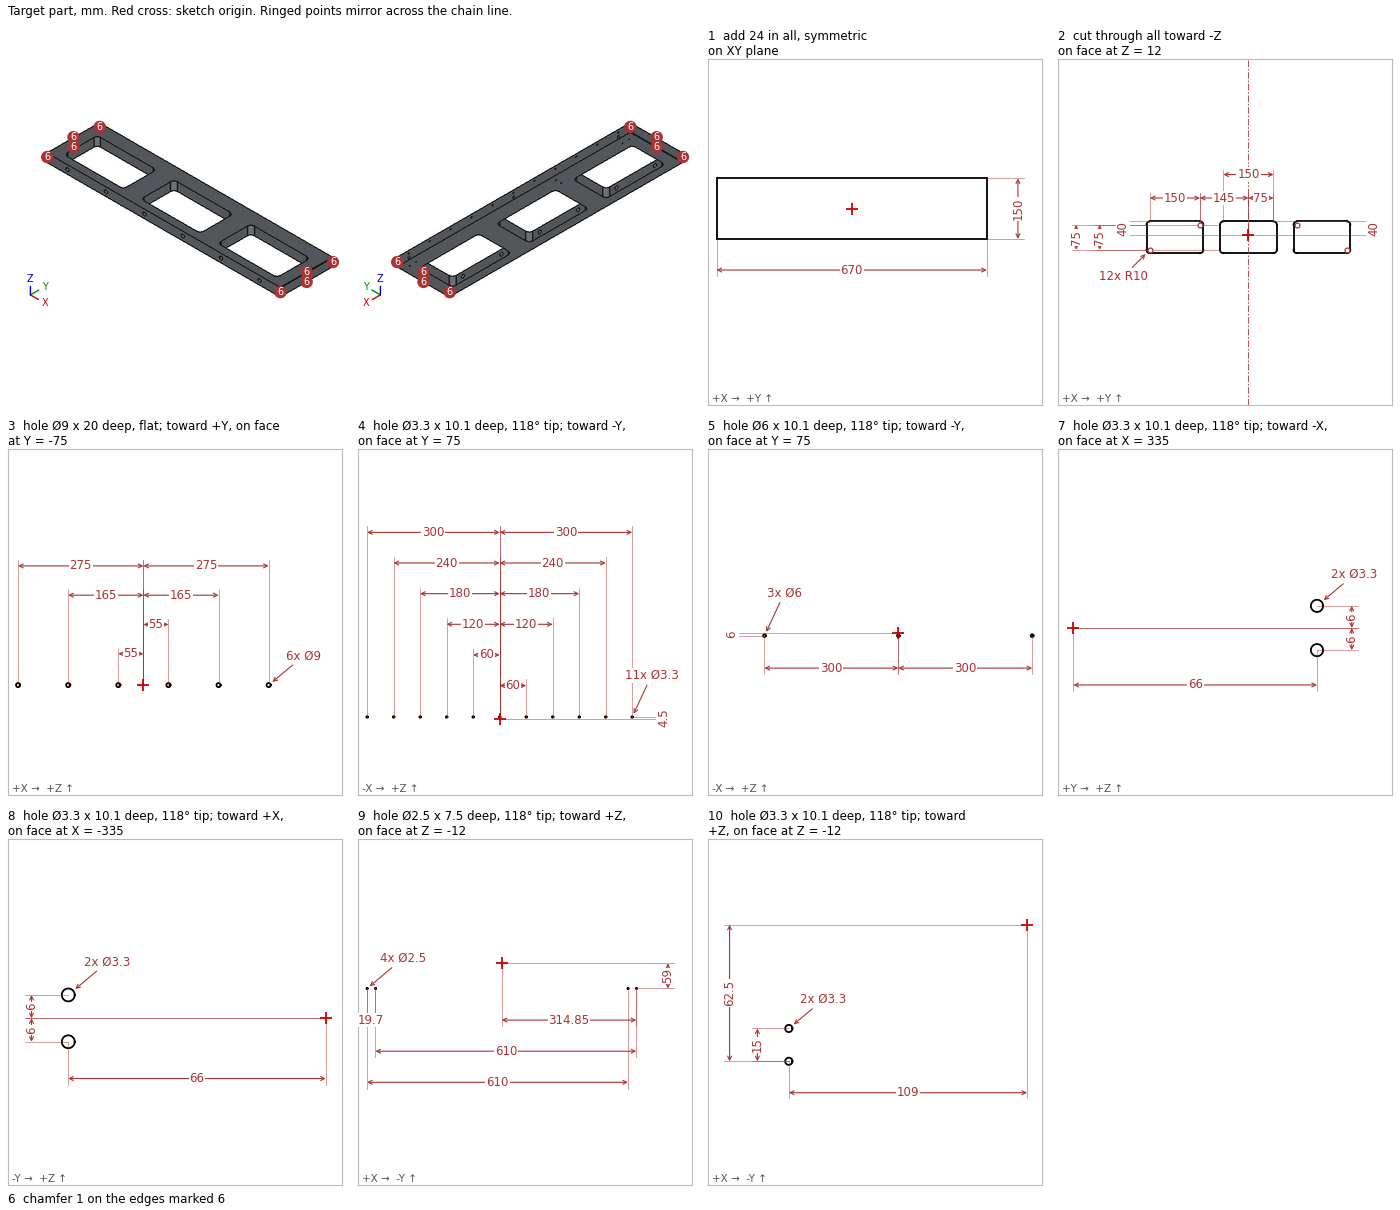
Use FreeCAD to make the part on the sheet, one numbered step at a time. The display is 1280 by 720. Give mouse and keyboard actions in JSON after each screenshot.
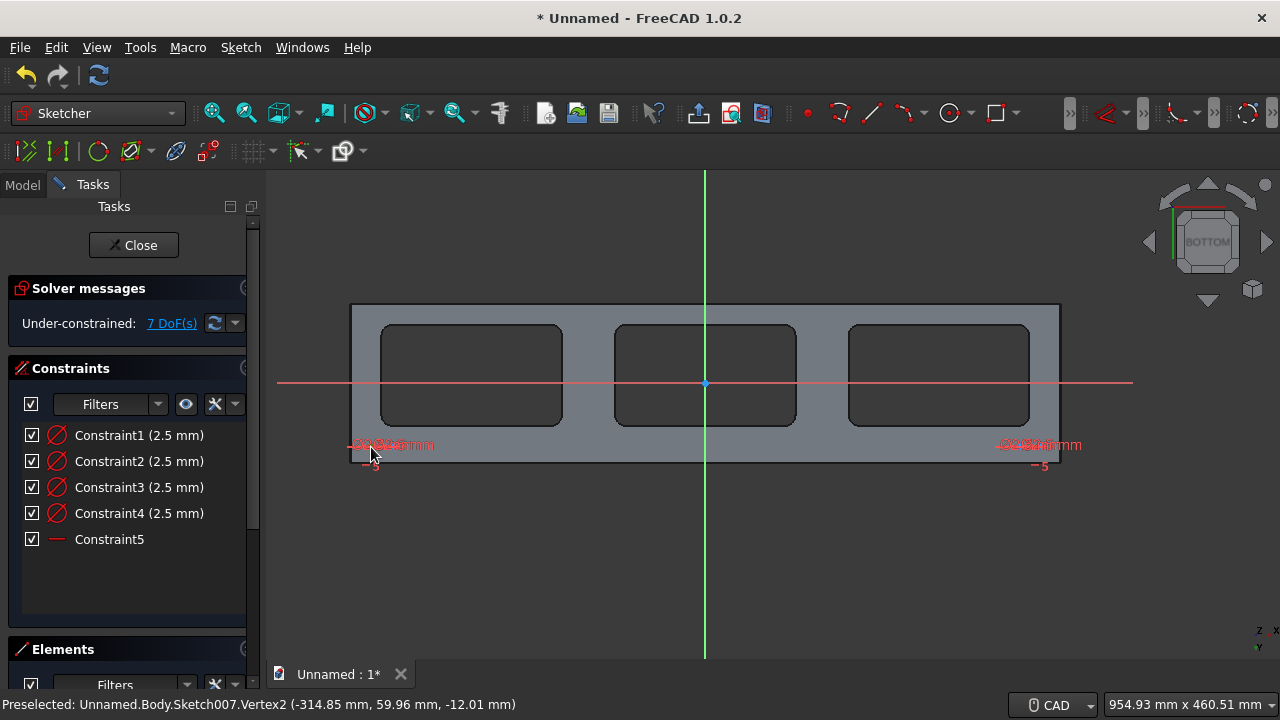
{"action": "left_click", "coordinate": [392, 447]}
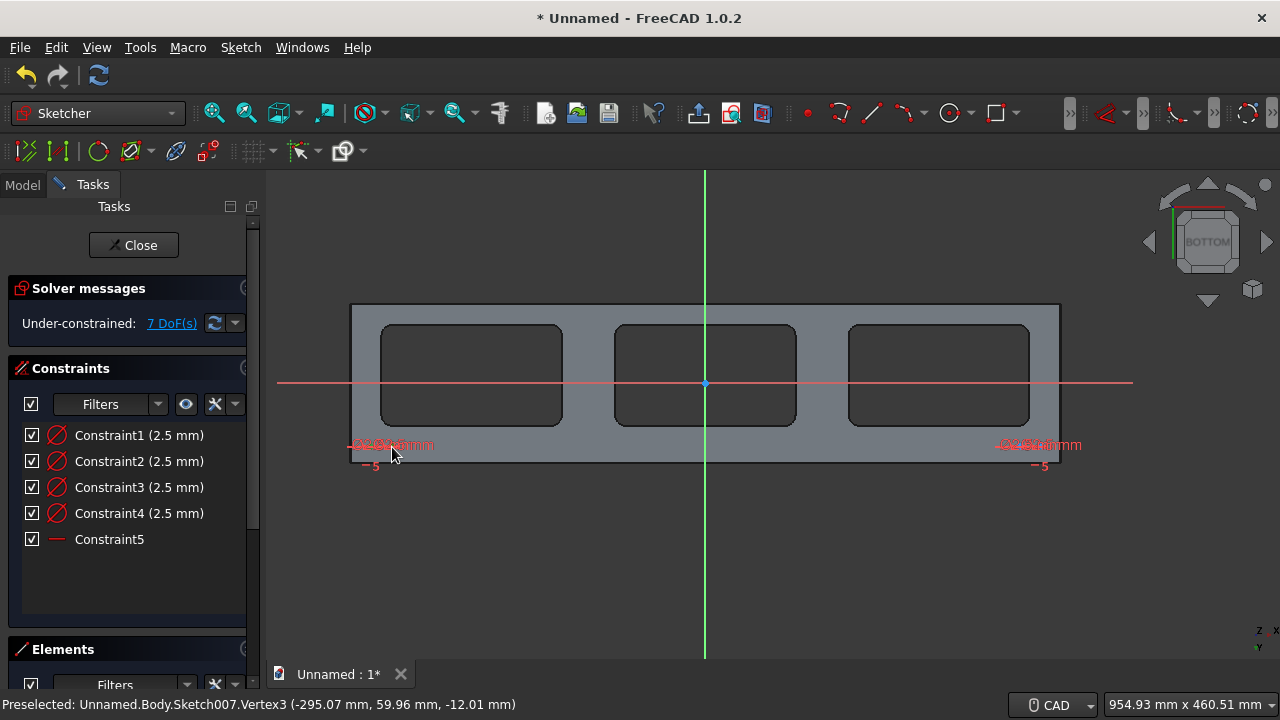
{"action": "key", "text": "h"}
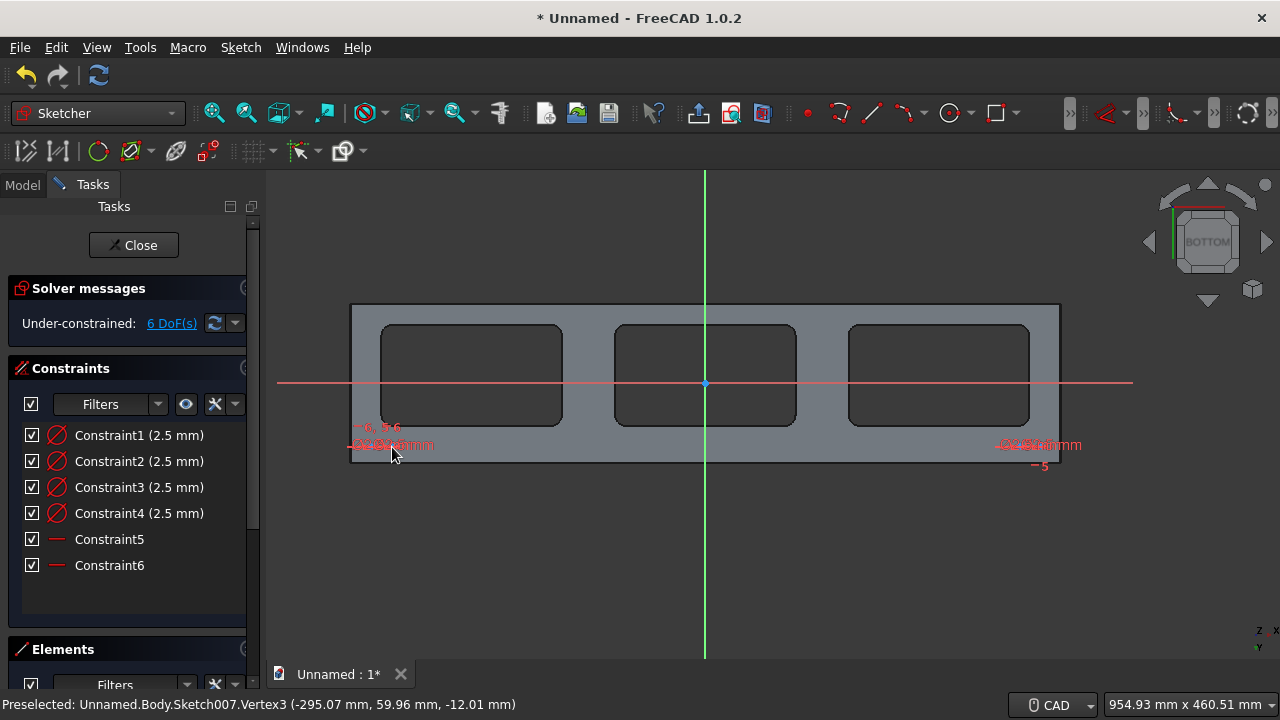
{"action": "left_click", "coordinate": [1040, 447]}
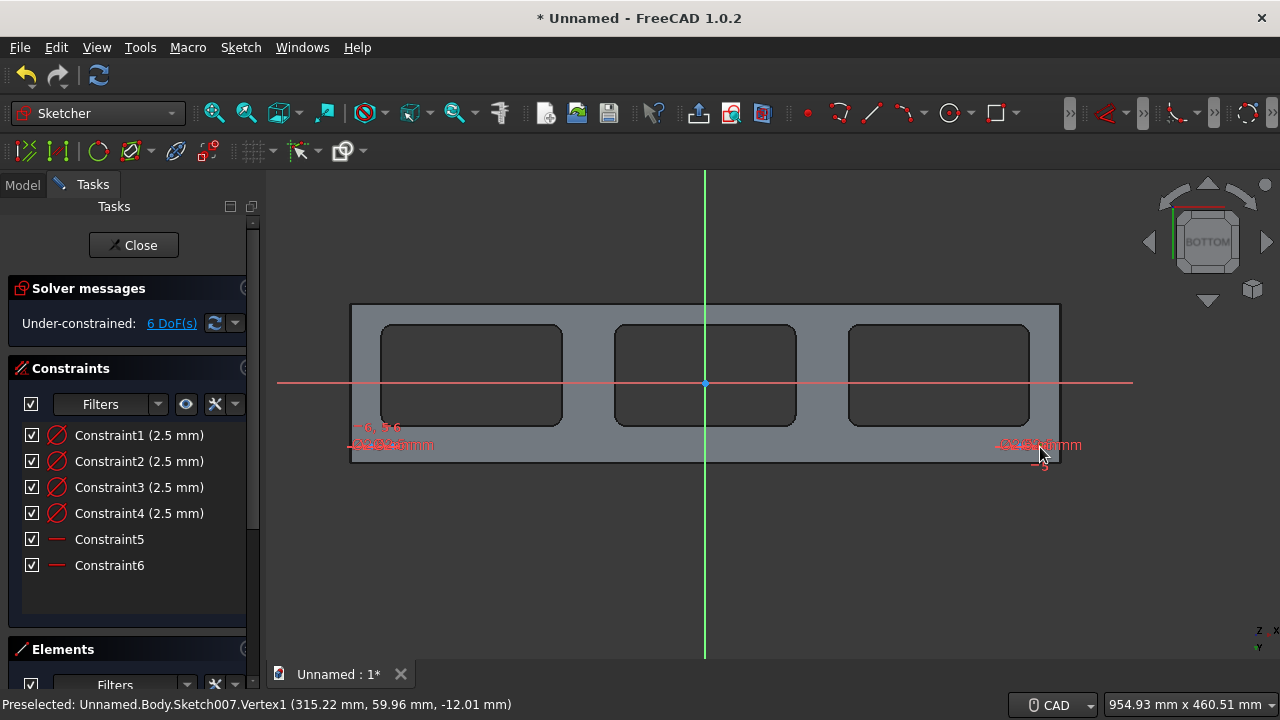
{"action": "left_click", "coordinate": [1019, 447]}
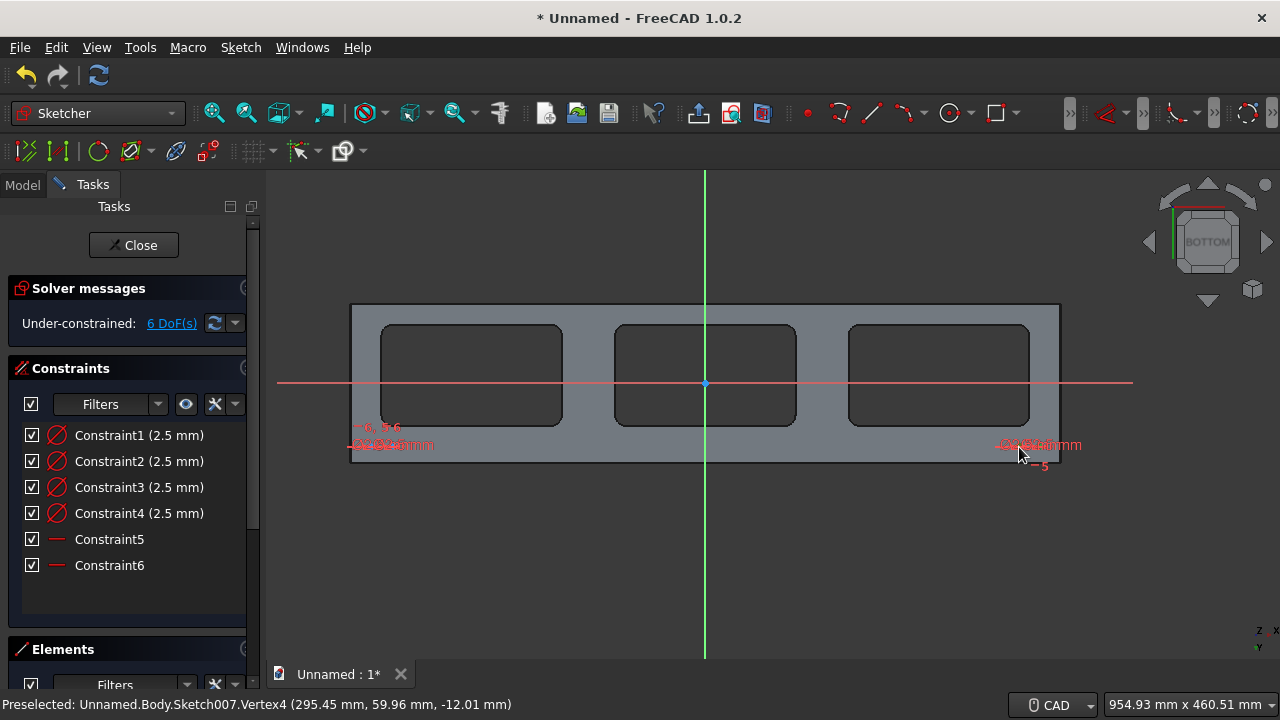
{"action": "key", "text": "h"}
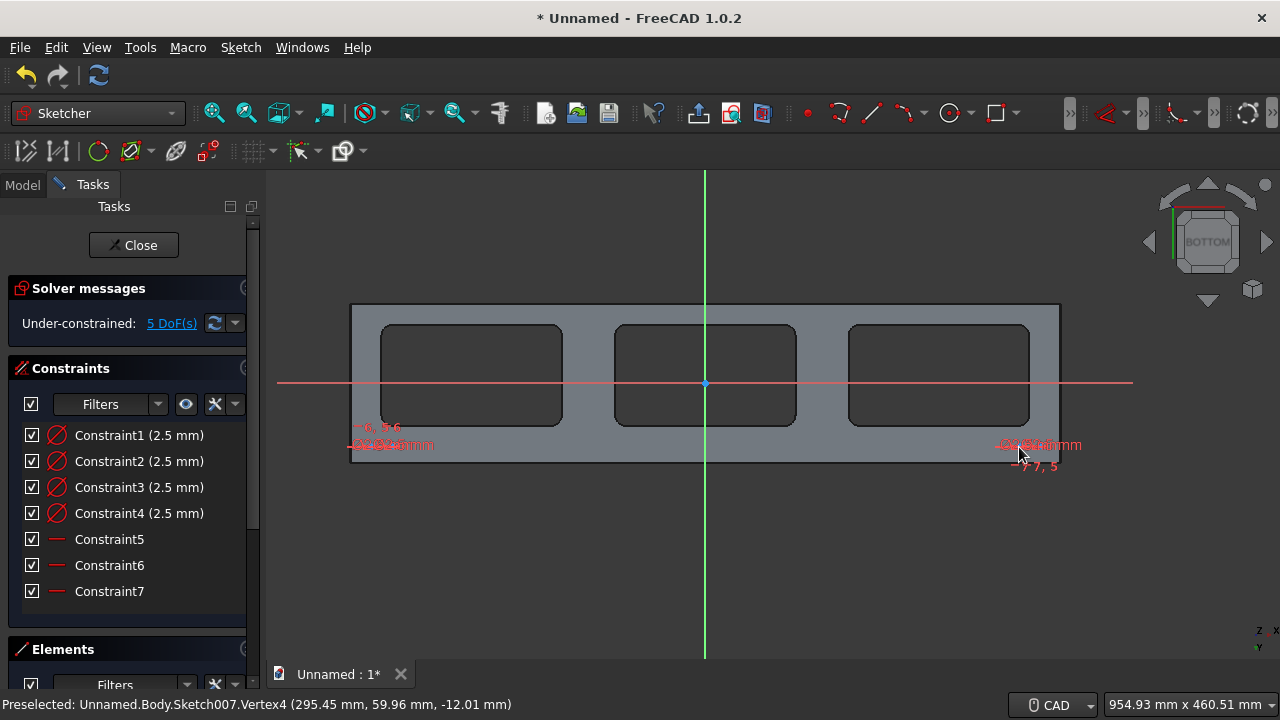
{"action": "left_click", "coordinate": [1106, 114]}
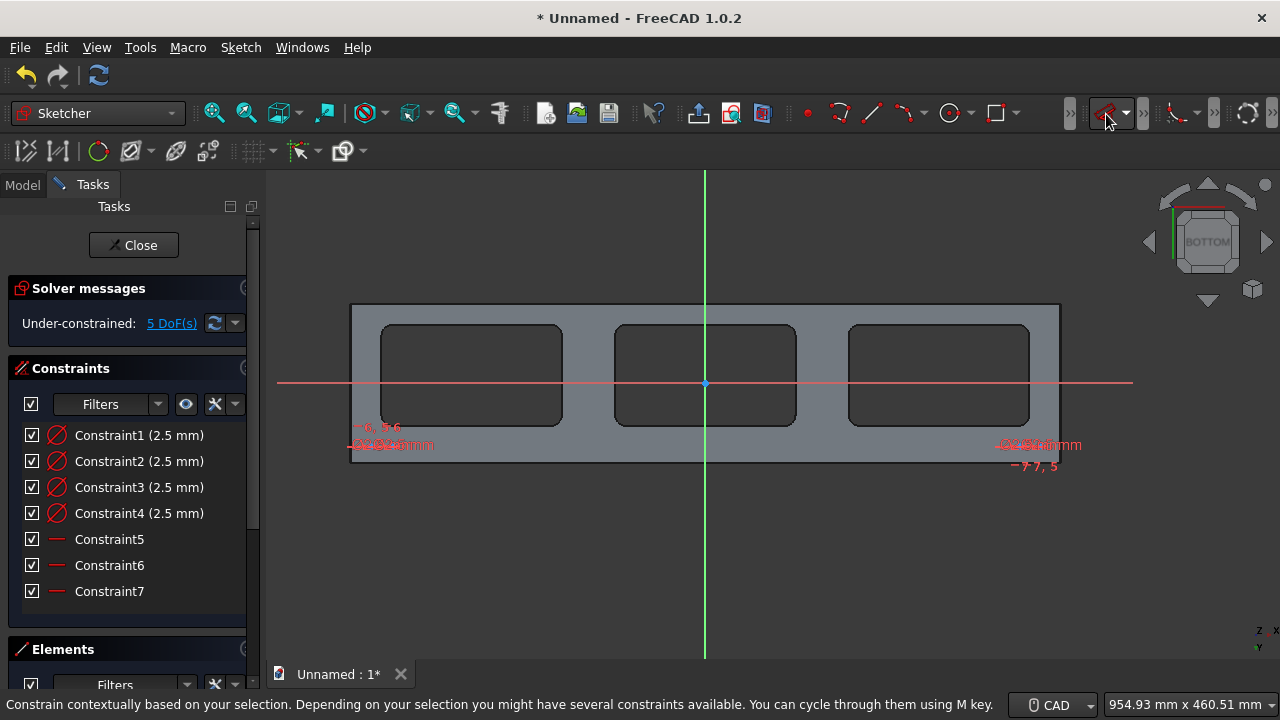
{"action": "left_click", "coordinate": [1040, 447]}
{"action": "left_click", "coordinate": [1074, 415]}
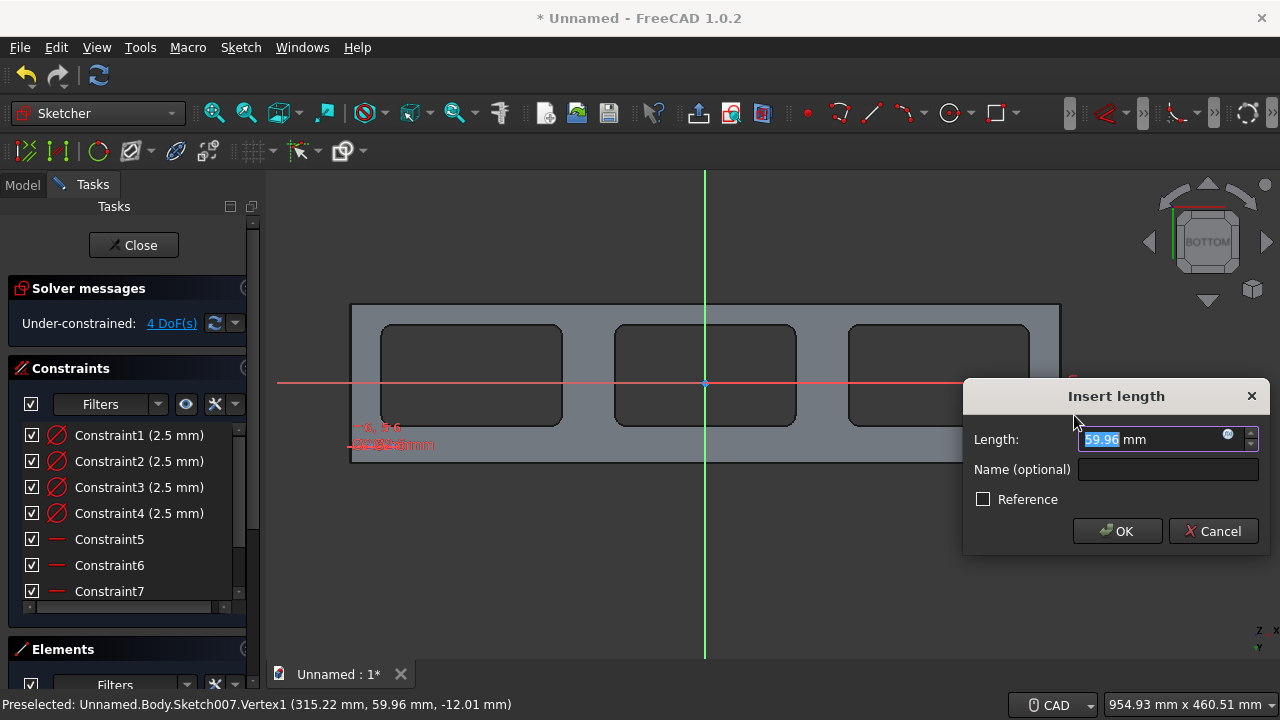
{"action": "type", "text": "59"}
{"action": "key", "text": "Return"}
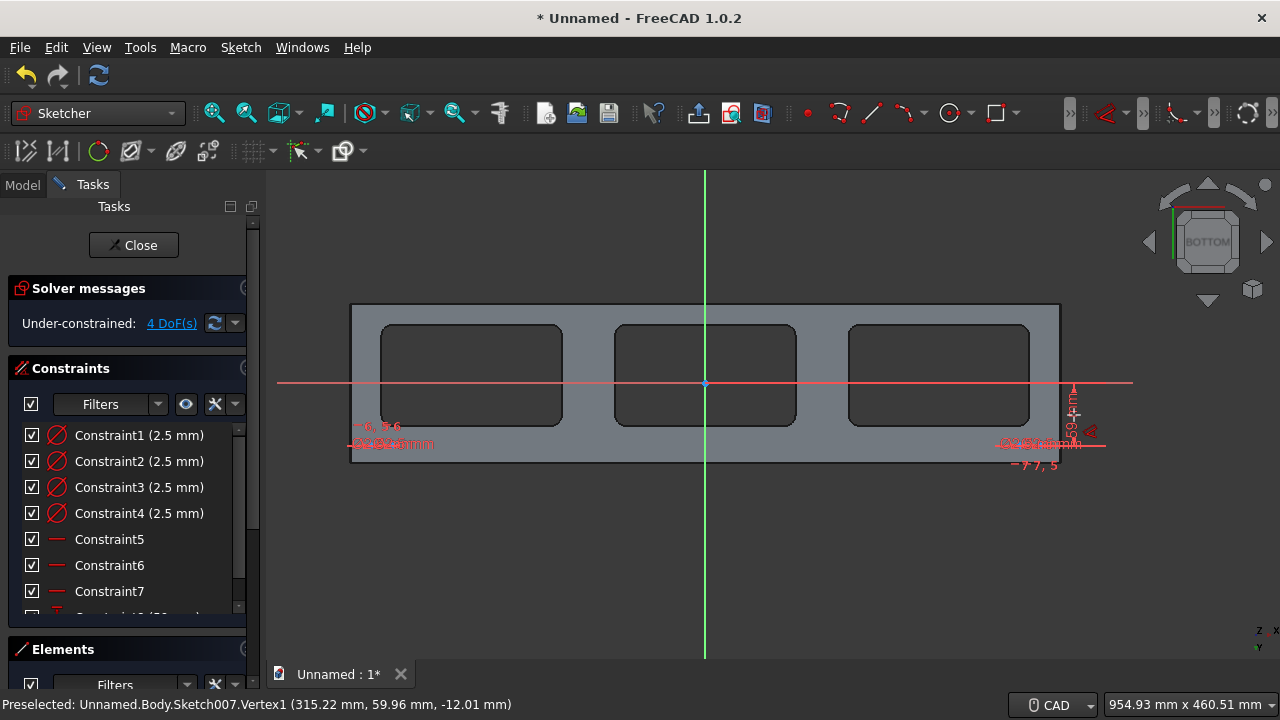
{"action": "left_click", "coordinate": [1040, 446]}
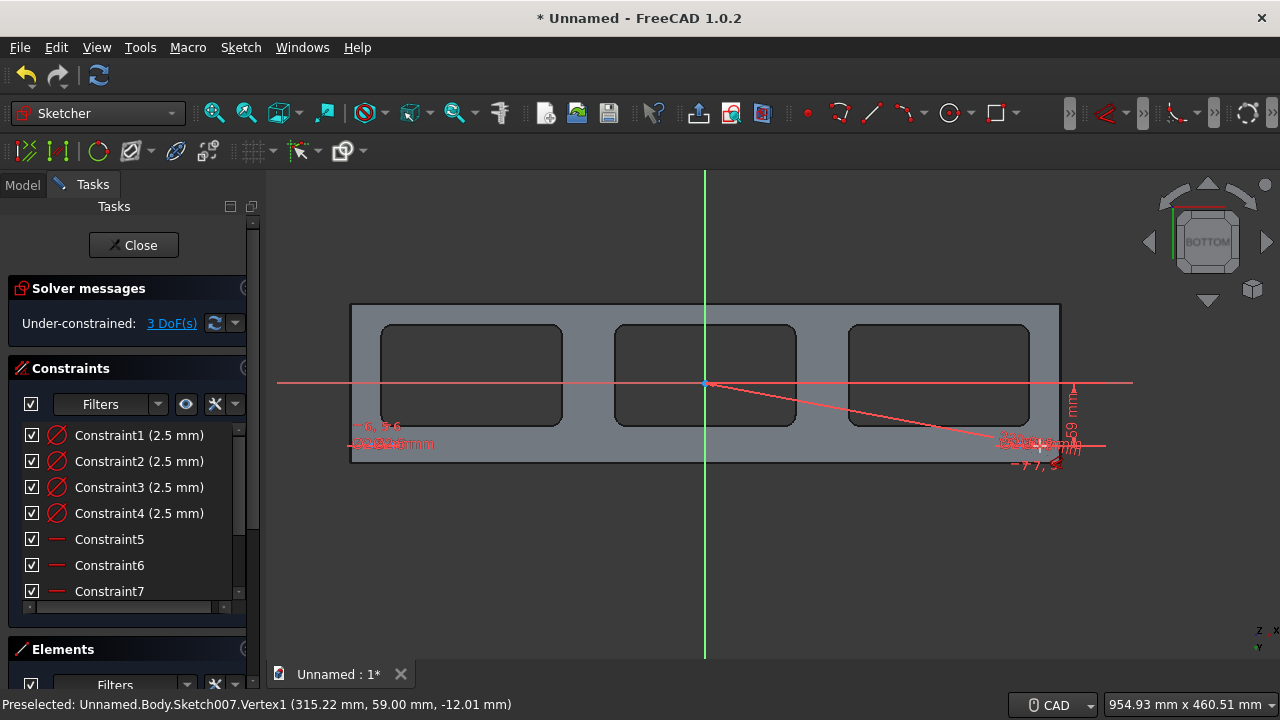
{"action": "left_click", "coordinate": [392, 446]}
{"action": "left_click", "coordinate": [567, 480]}